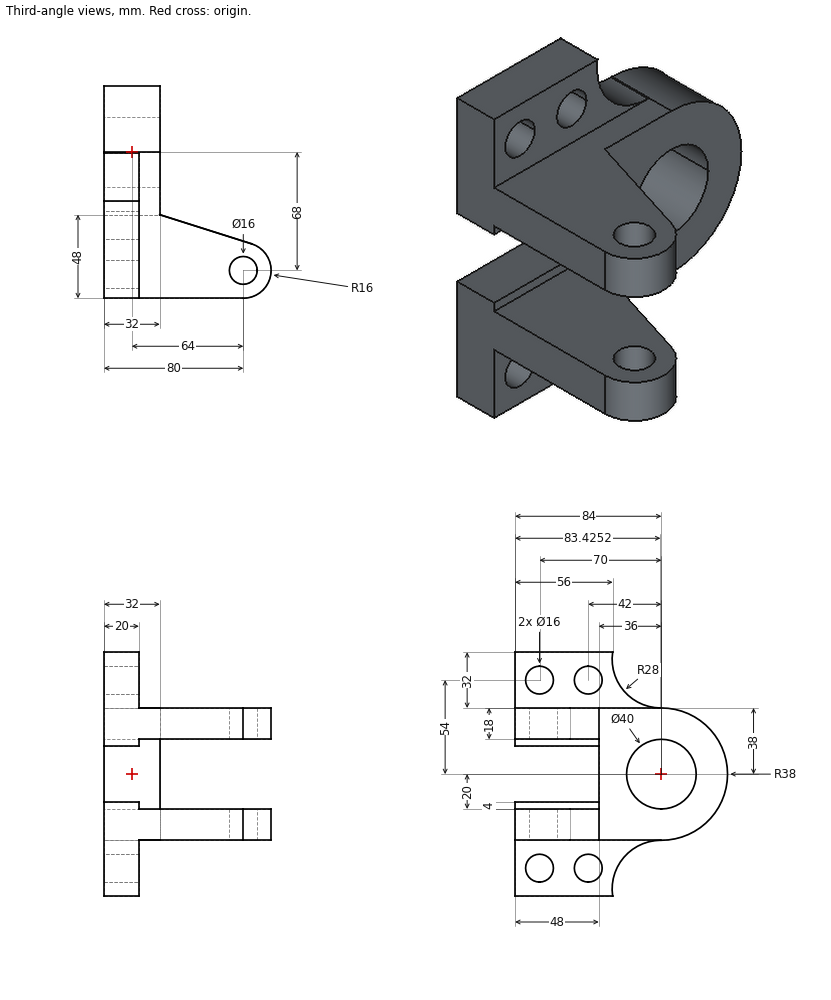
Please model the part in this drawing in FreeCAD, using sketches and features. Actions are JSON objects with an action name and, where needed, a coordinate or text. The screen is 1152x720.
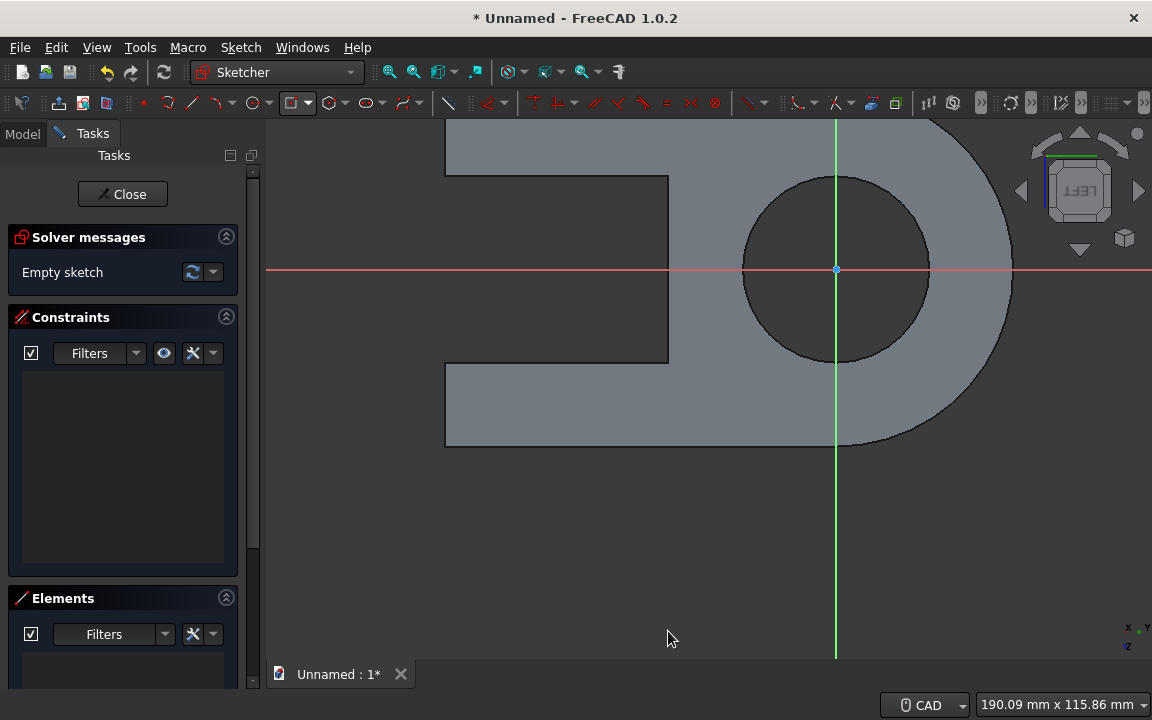
{"action": "left_click", "coordinate": [168, 104]}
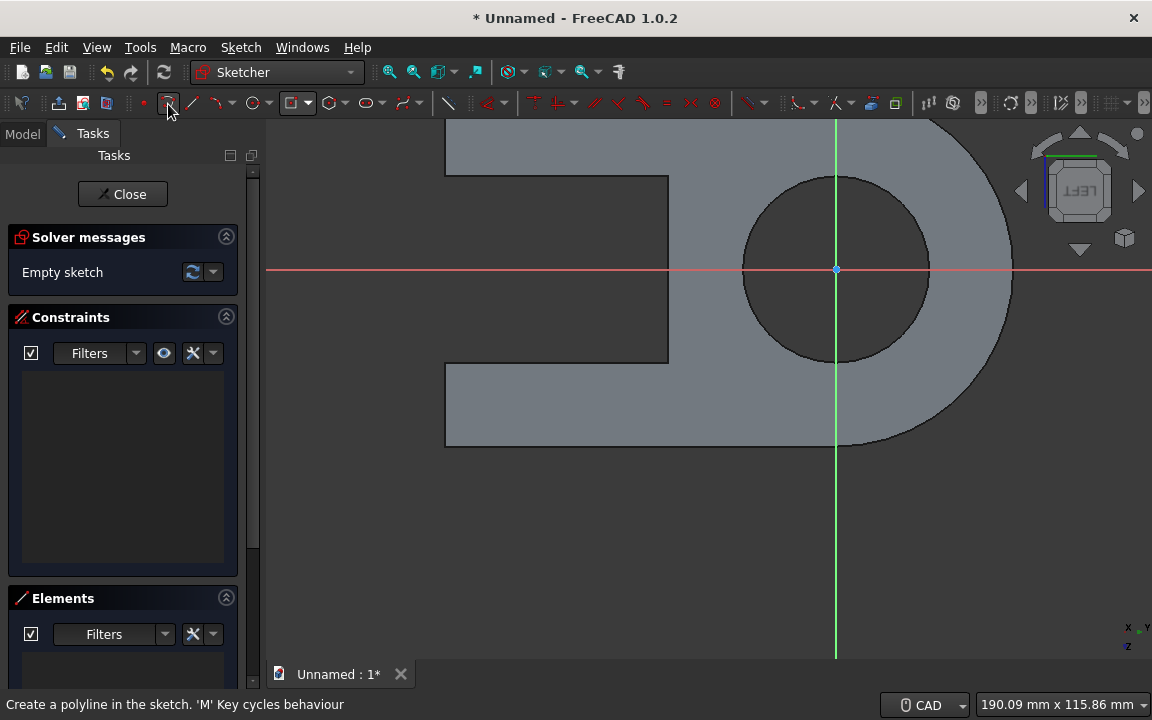
{"action": "scroll", "coordinate": [833, 447], "scroll_direction": "up", "scroll_amount": 9}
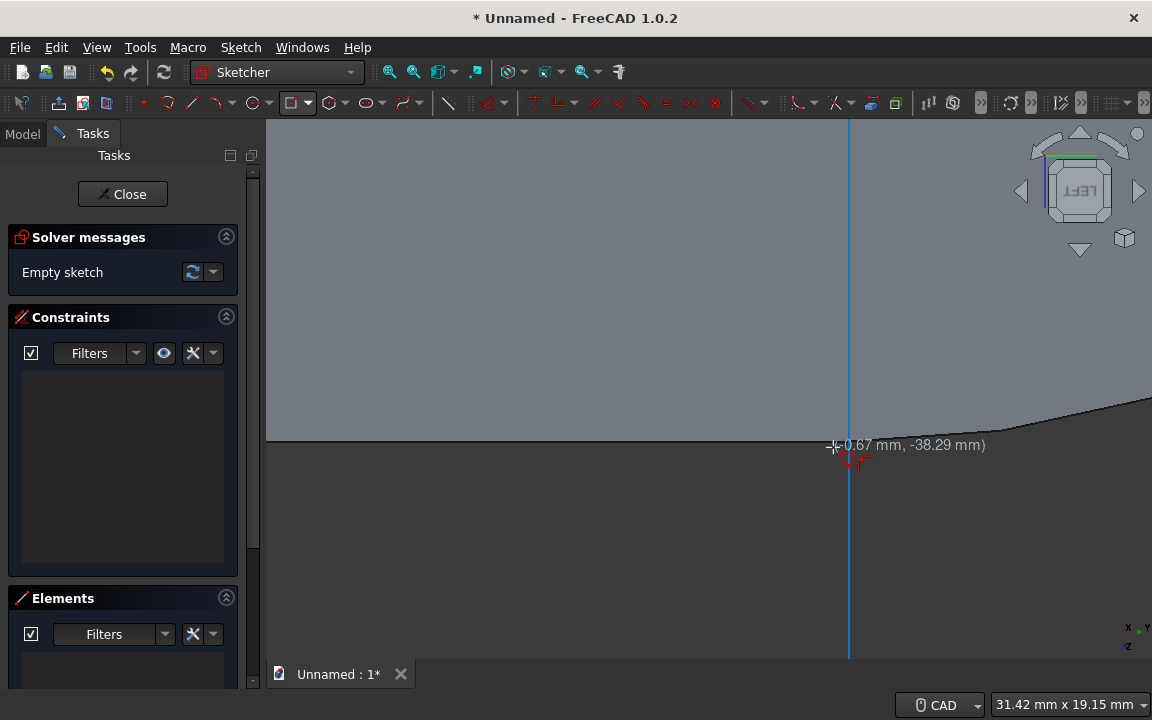
{"action": "left_click", "coordinate": [833, 442]}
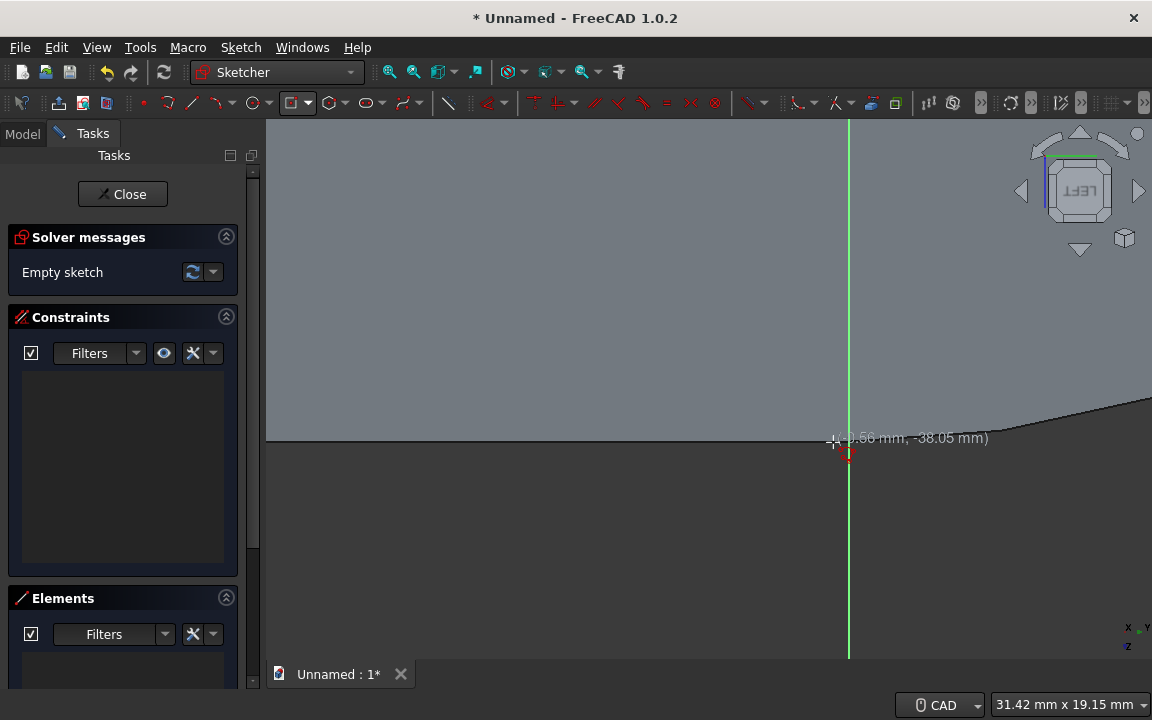
{"action": "scroll", "coordinate": [834, 395], "scroll_direction": "down", "scroll_amount": 9}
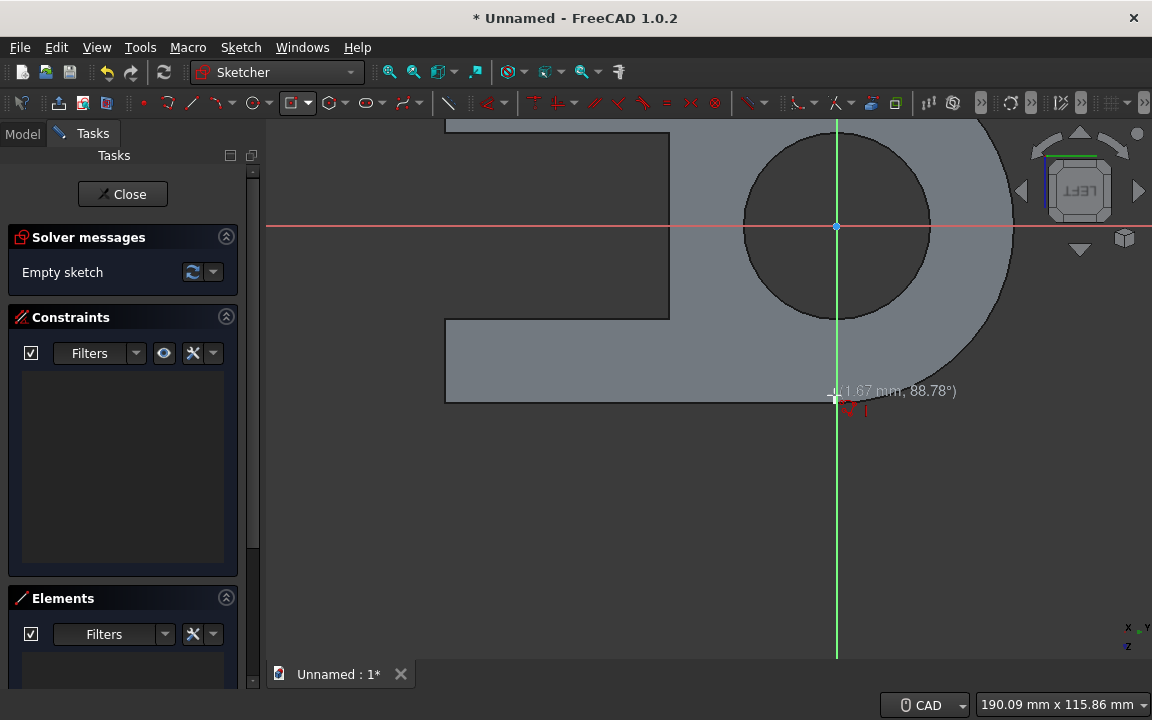
{"action": "left_click", "coordinate": [445, 403]}
{"action": "left_click", "coordinate": [445, 552]}
{"action": "left_click", "coordinate": [706, 552]}
{"action": "right_click", "coordinate": [706, 552]}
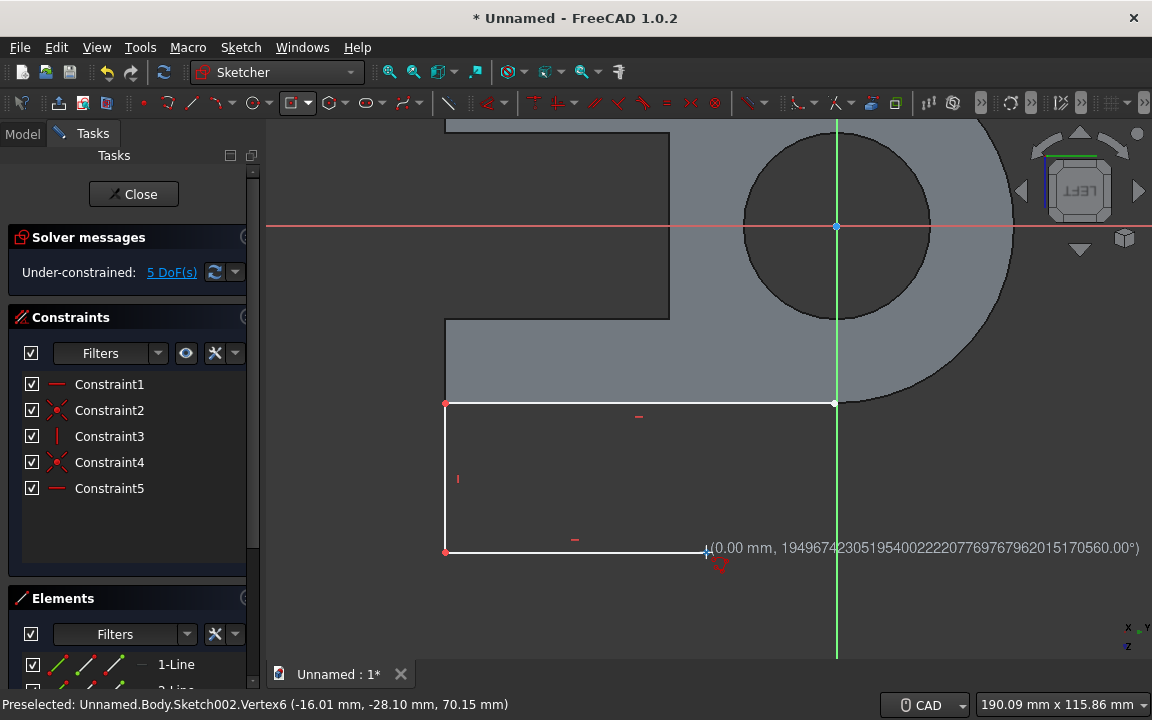
{"action": "left_click", "coordinate": [216, 104]}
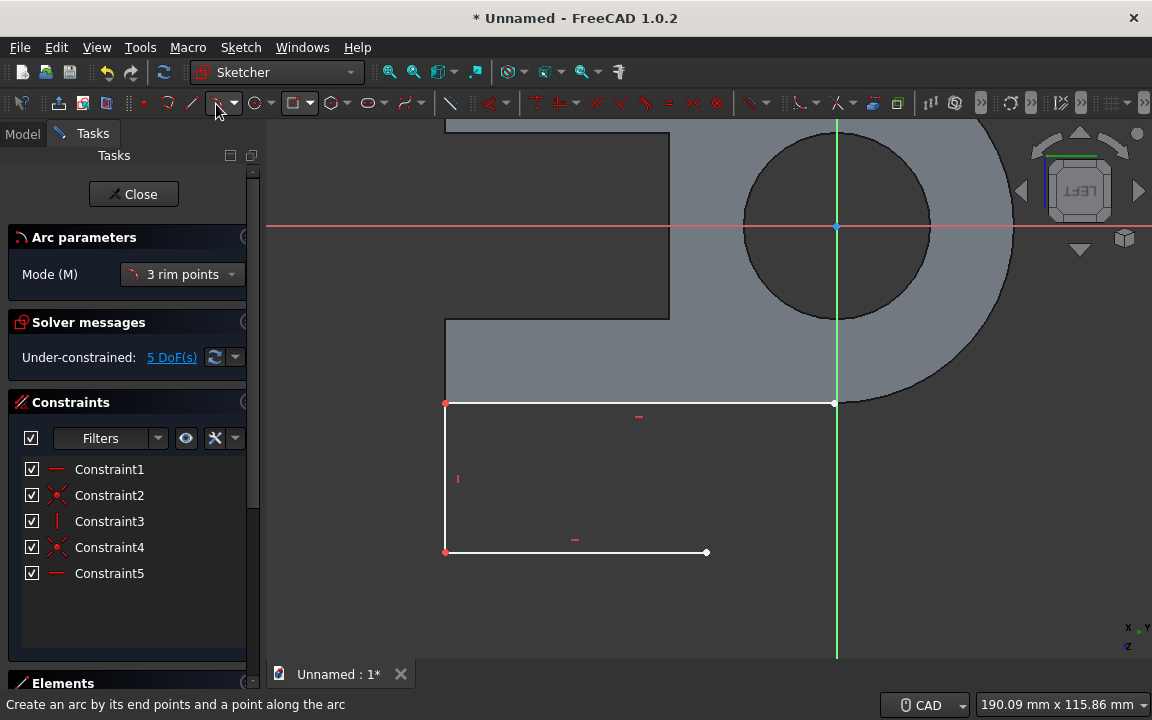
{"action": "left_click", "coordinate": [706, 553]}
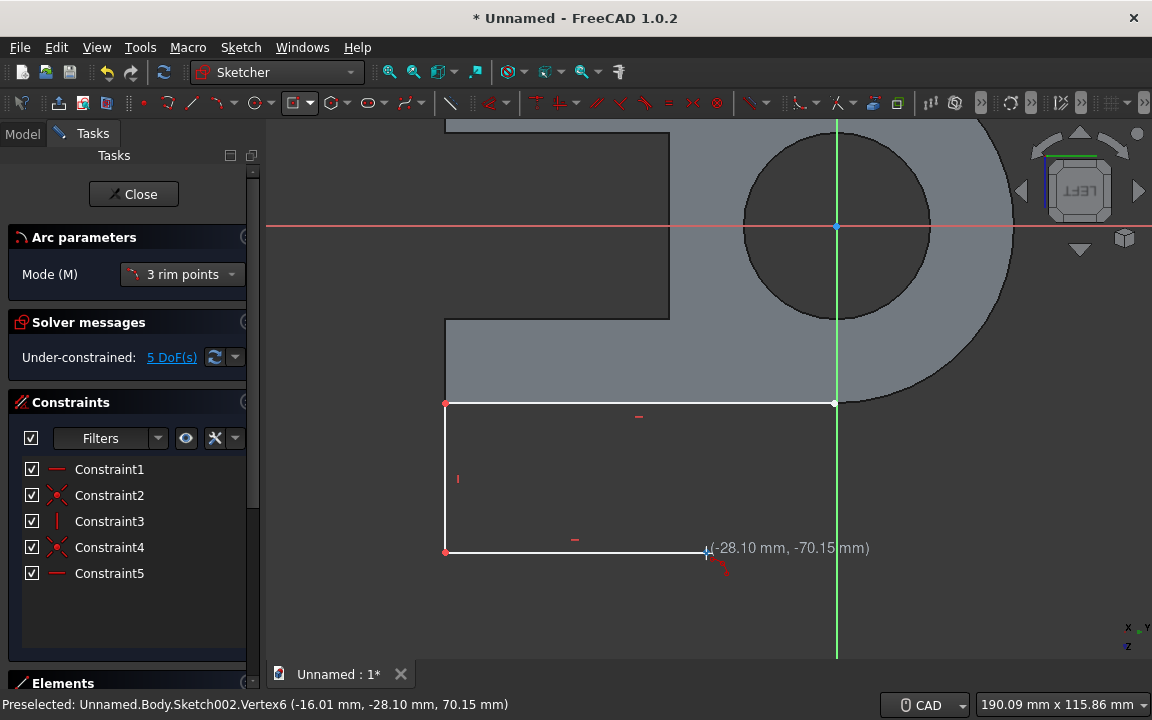
{"action": "scroll", "coordinate": [834, 403], "scroll_direction": "up", "scroll_amount": 9}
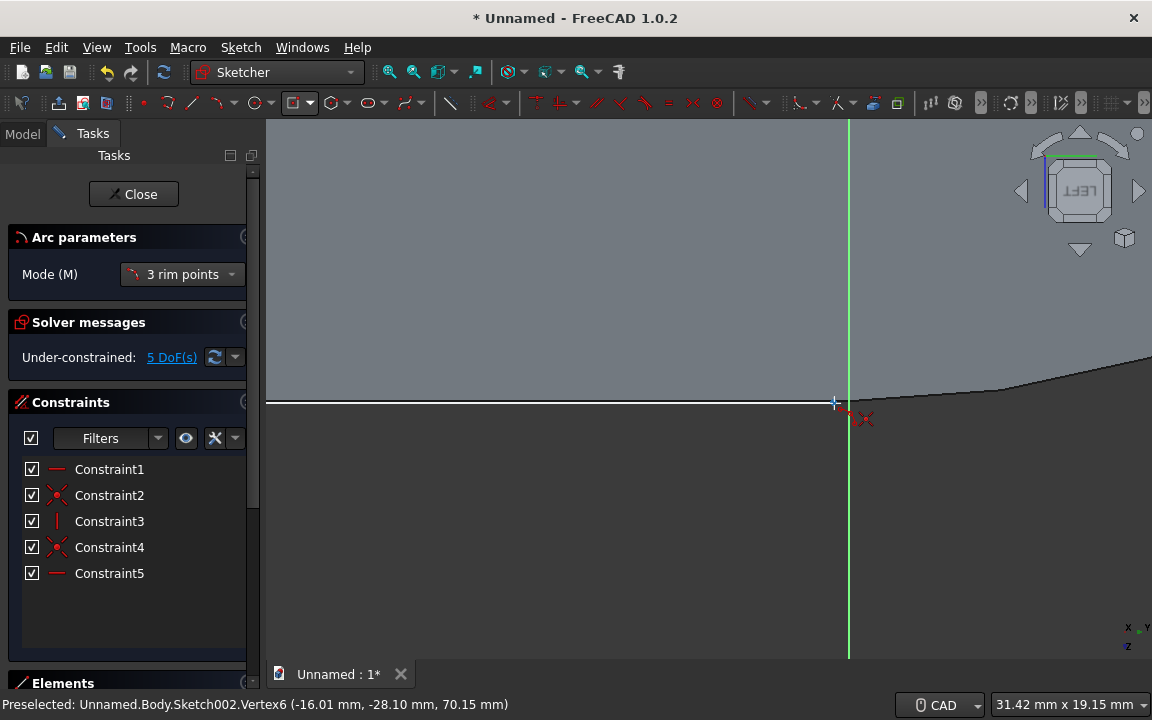
{"action": "left_click", "coordinate": [833, 403]}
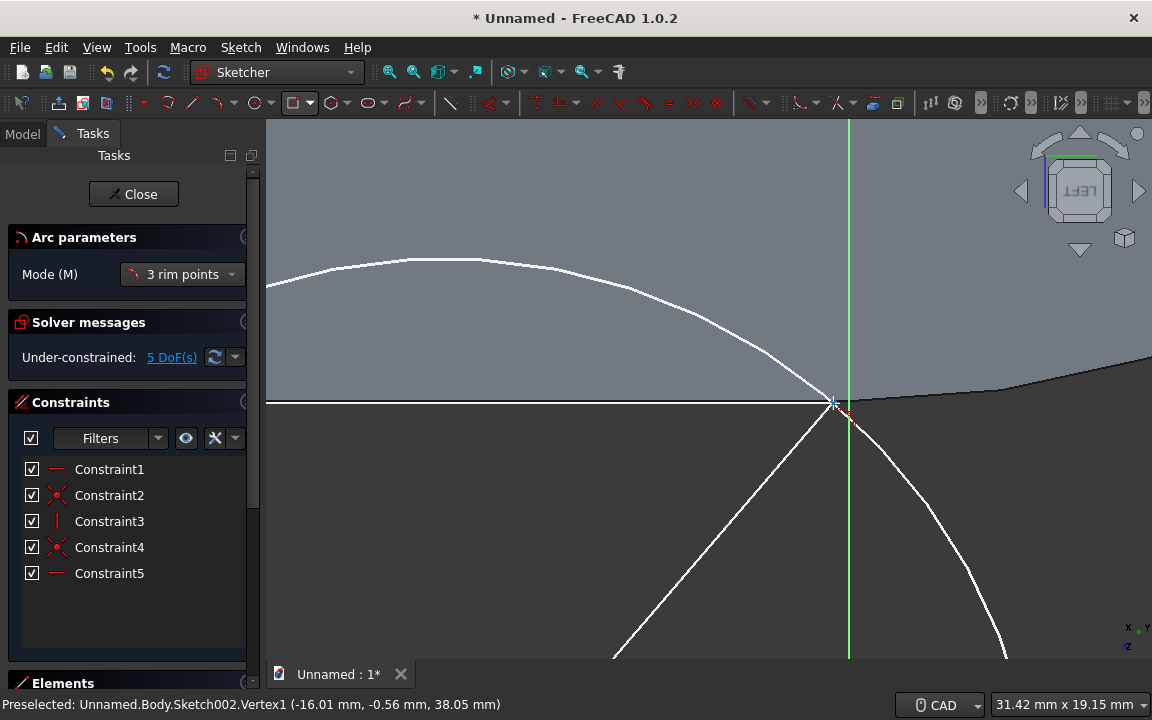
{"action": "scroll", "coordinate": [834, 403], "scroll_direction": "down", "scroll_amount": 9}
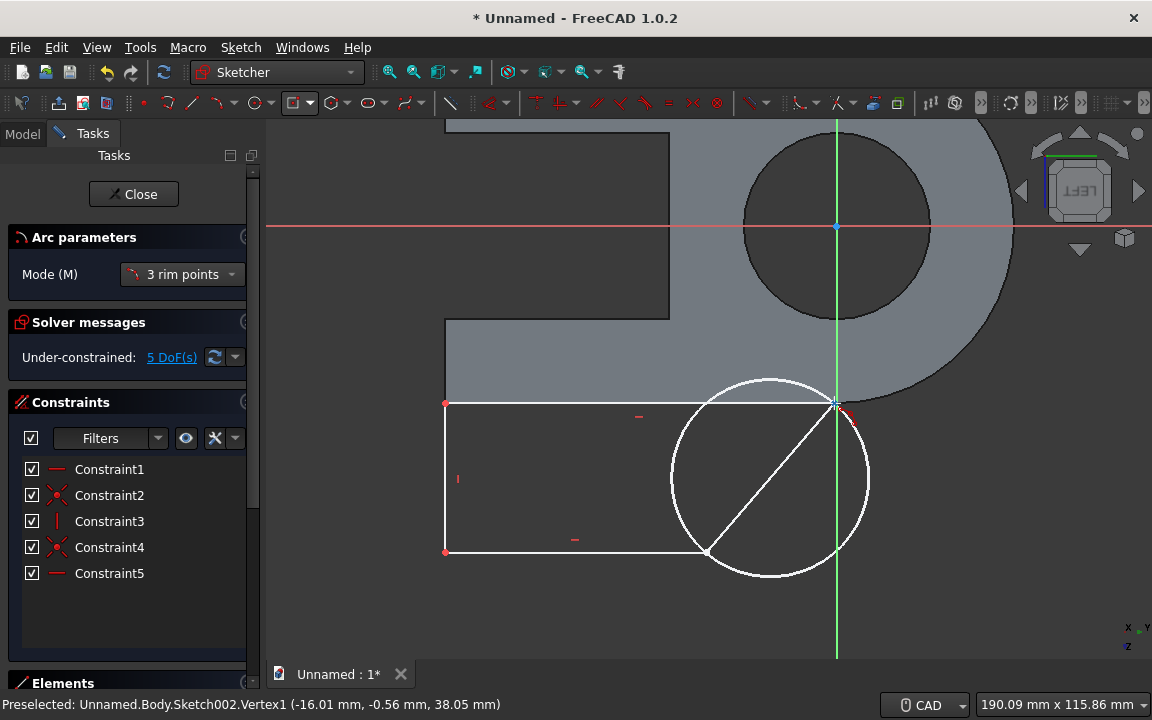
{"action": "left_click", "coordinate": [737, 449]}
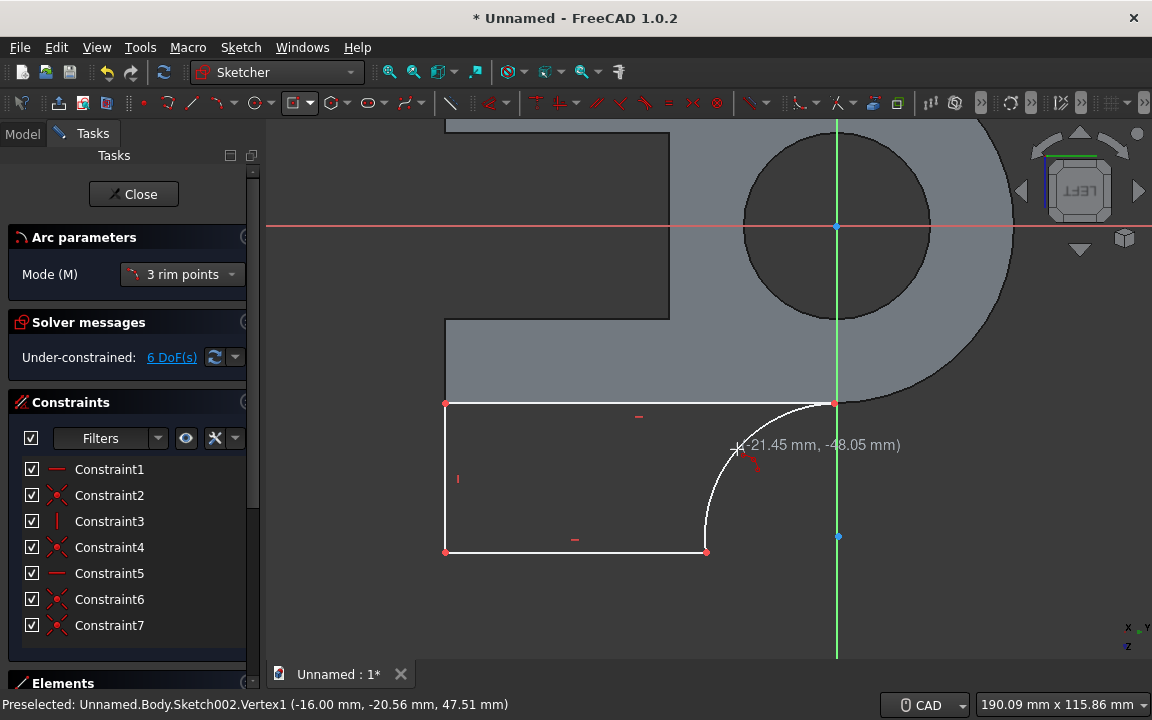
{"action": "left_click", "coordinate": [256, 104]}